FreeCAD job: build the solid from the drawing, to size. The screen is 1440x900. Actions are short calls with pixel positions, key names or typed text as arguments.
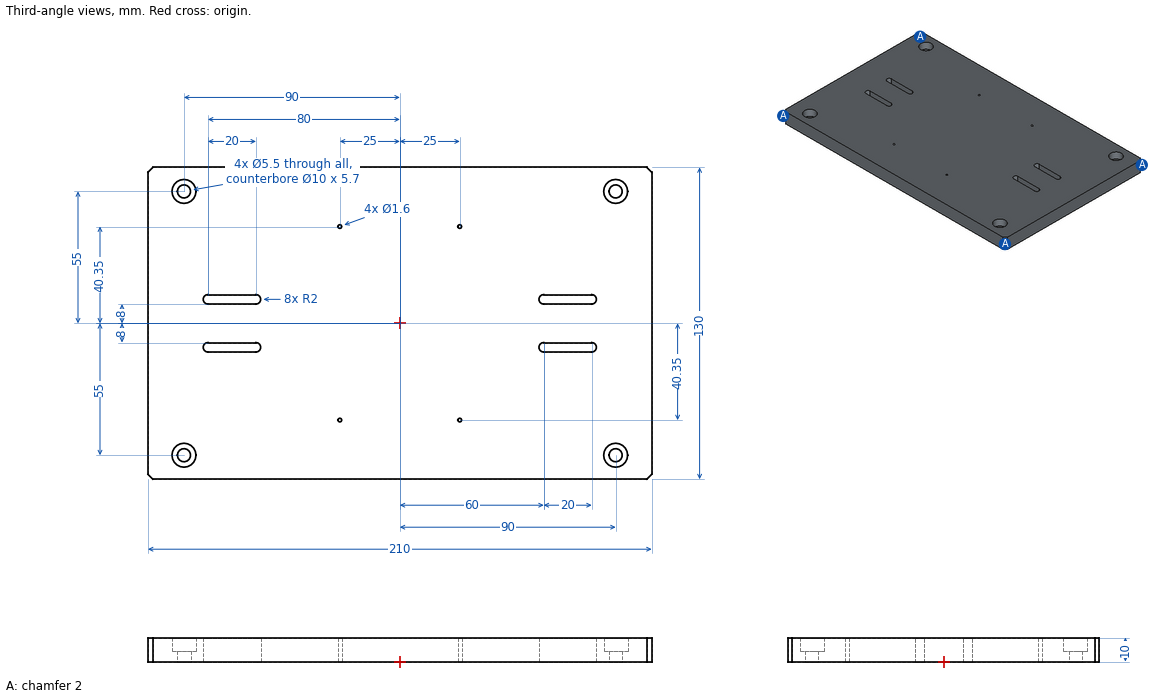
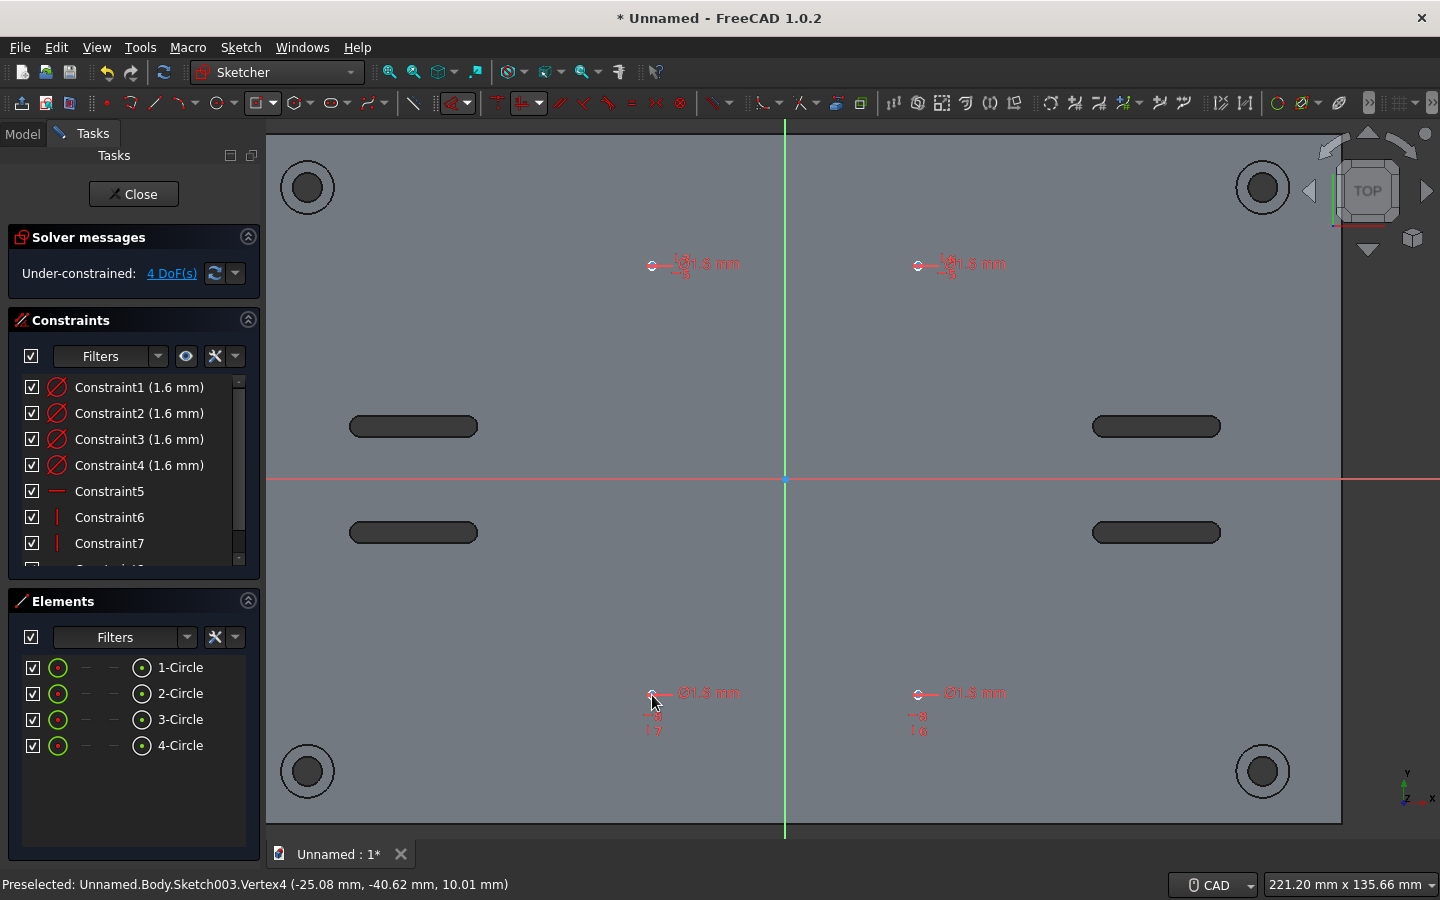
click(652, 266)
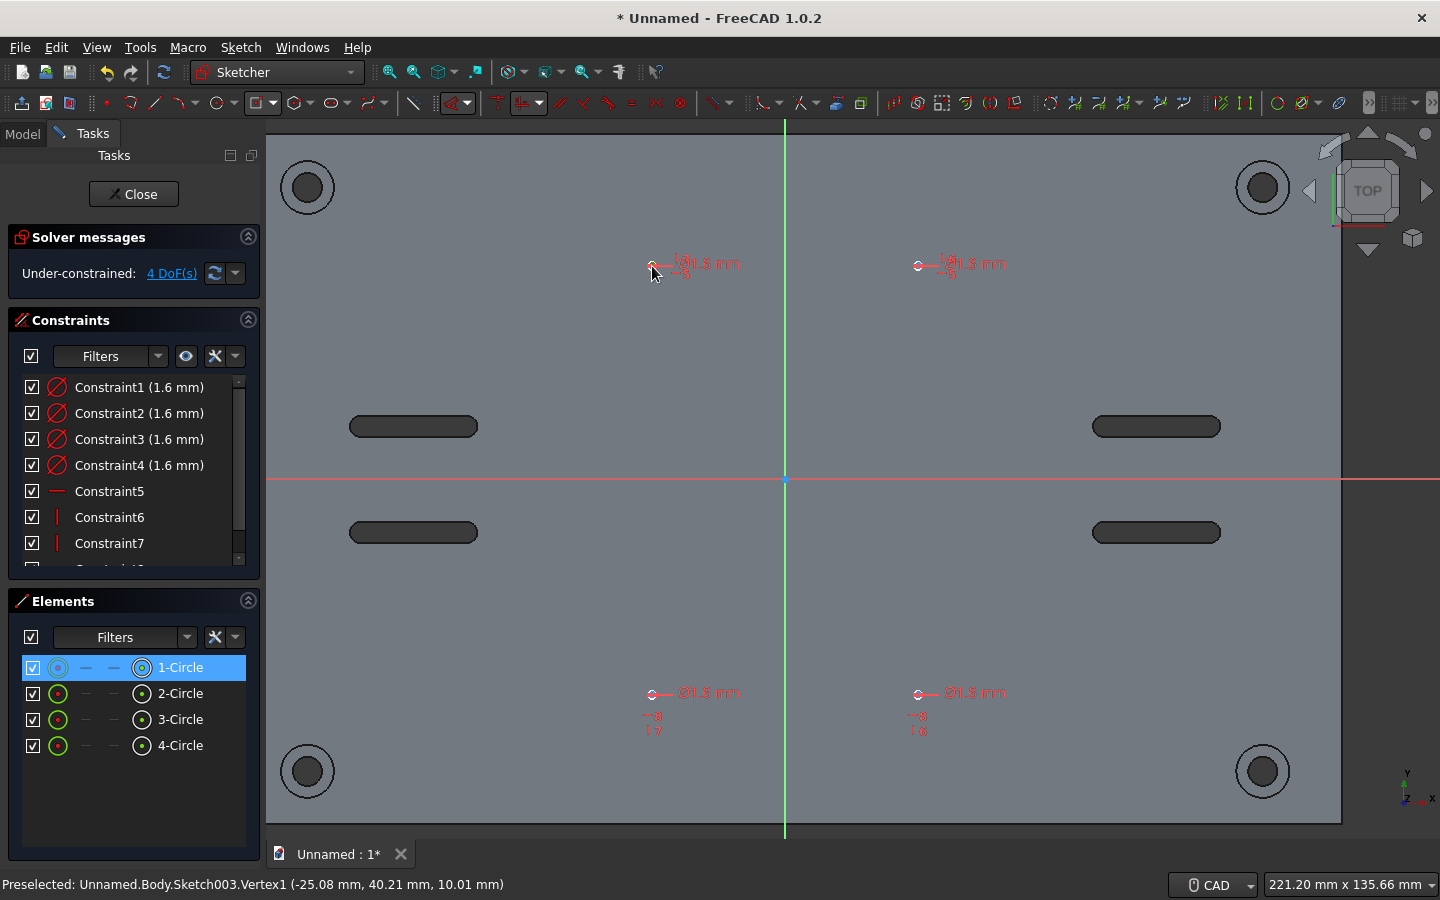
click(470, 104)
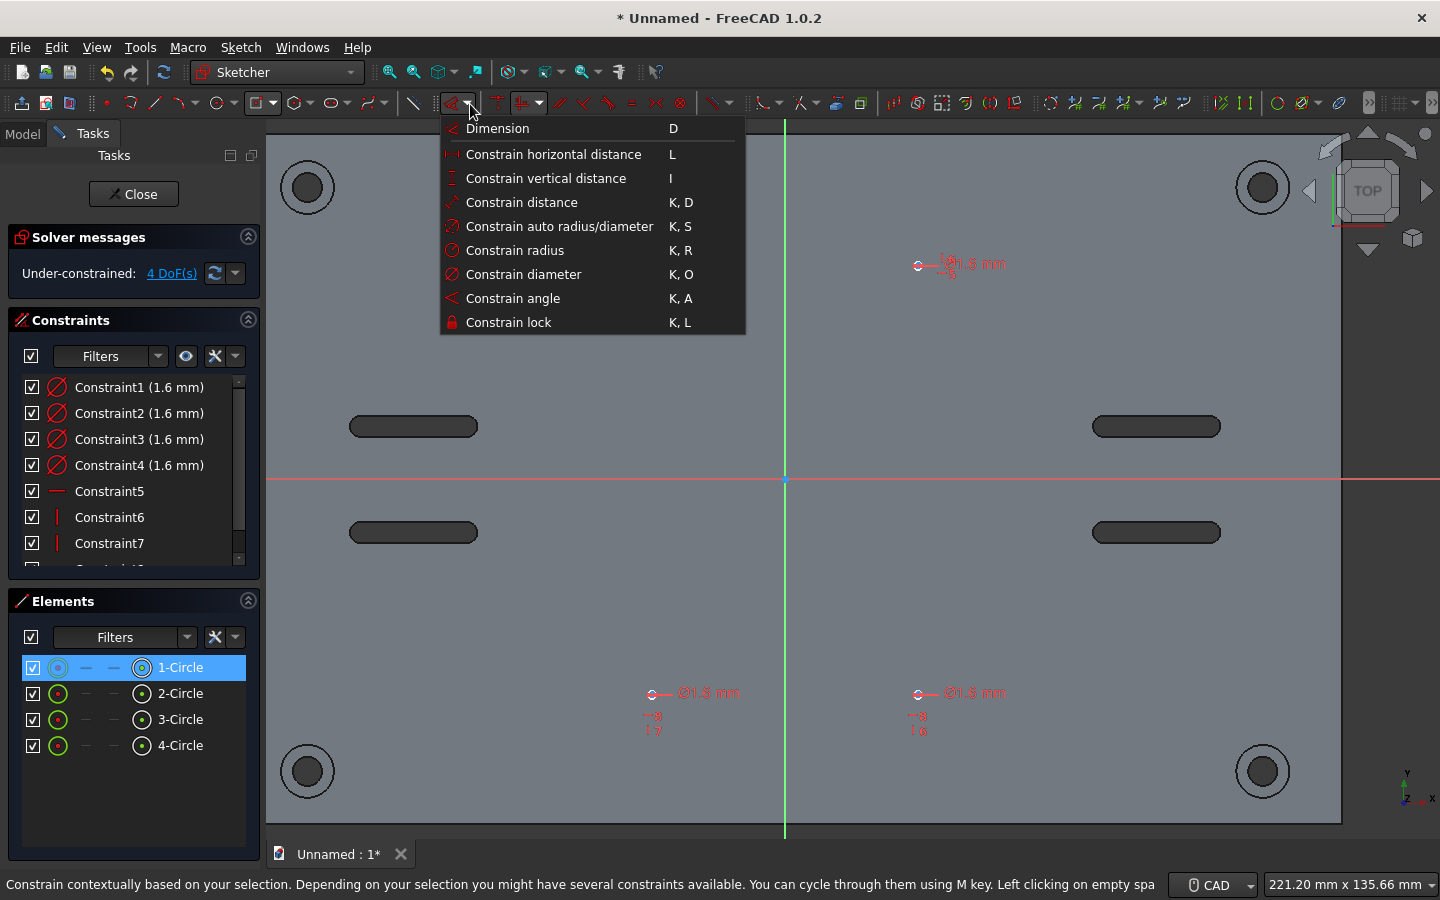
click(593, 154)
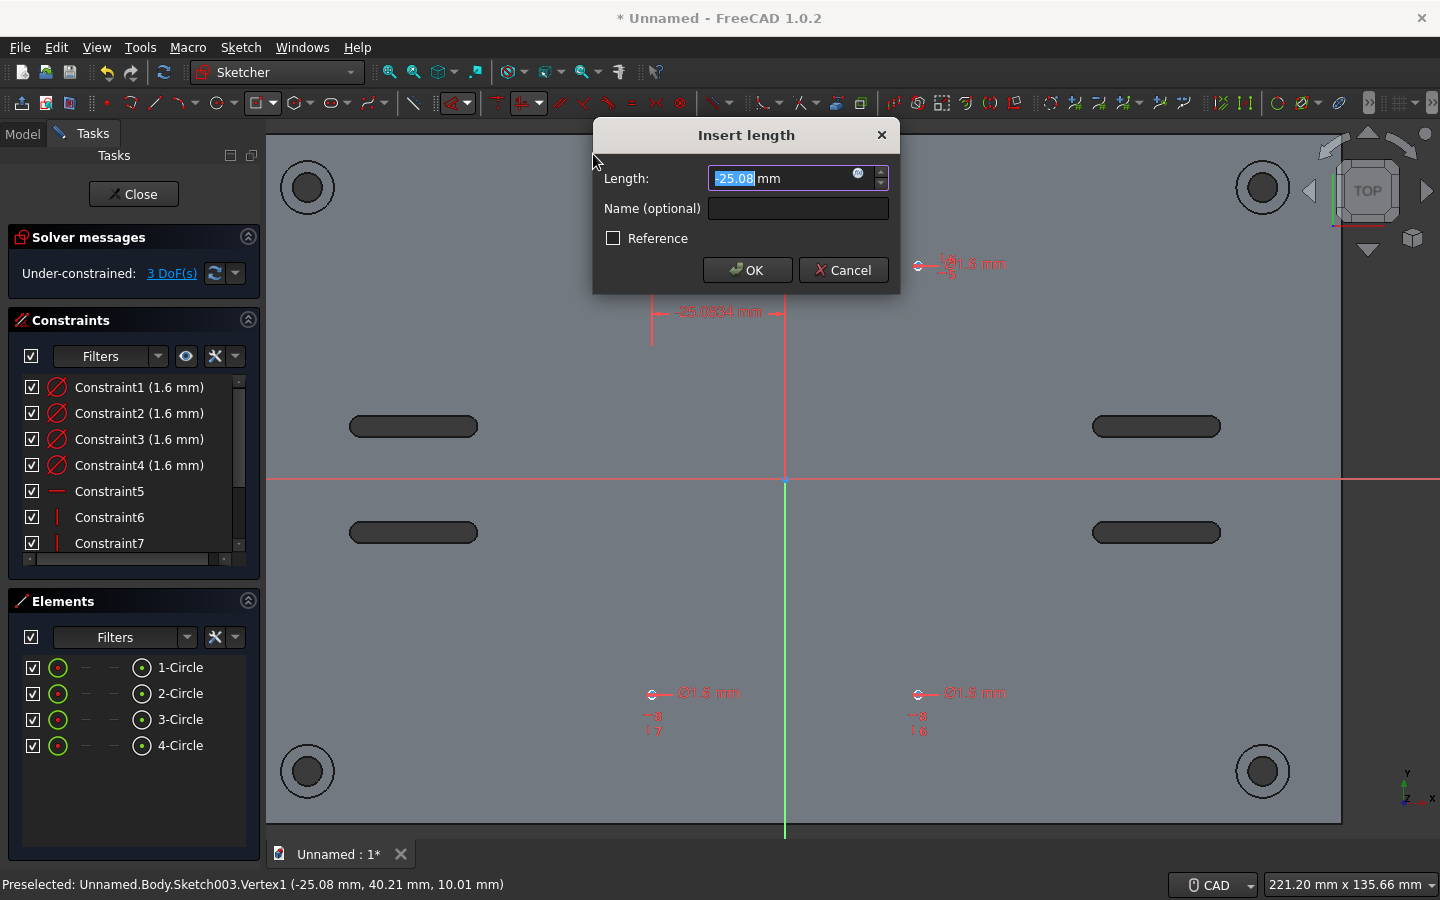
text(-25)
key(Return)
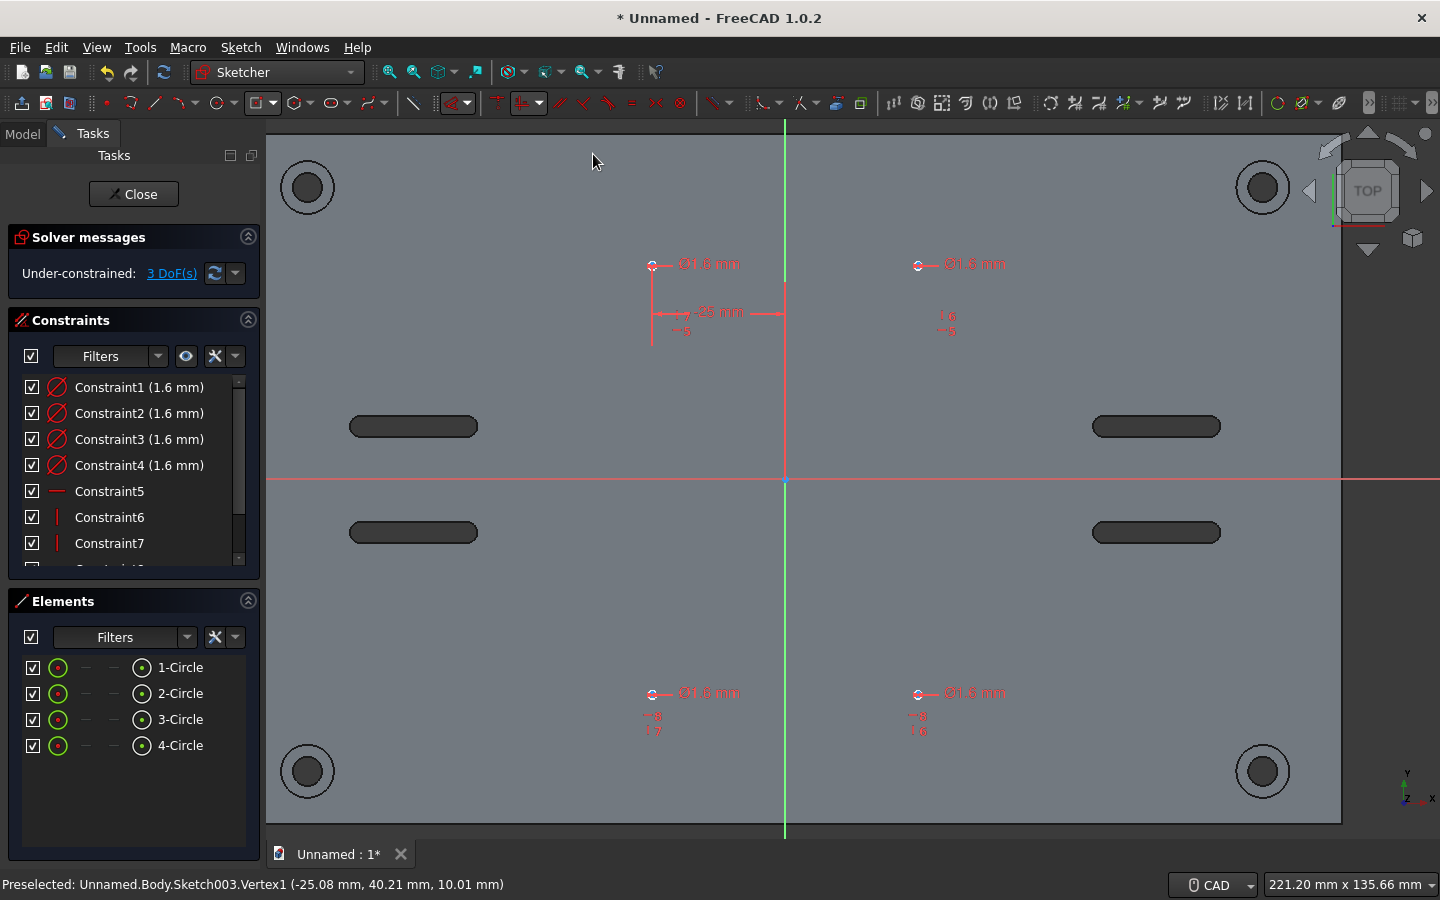
click(918, 266)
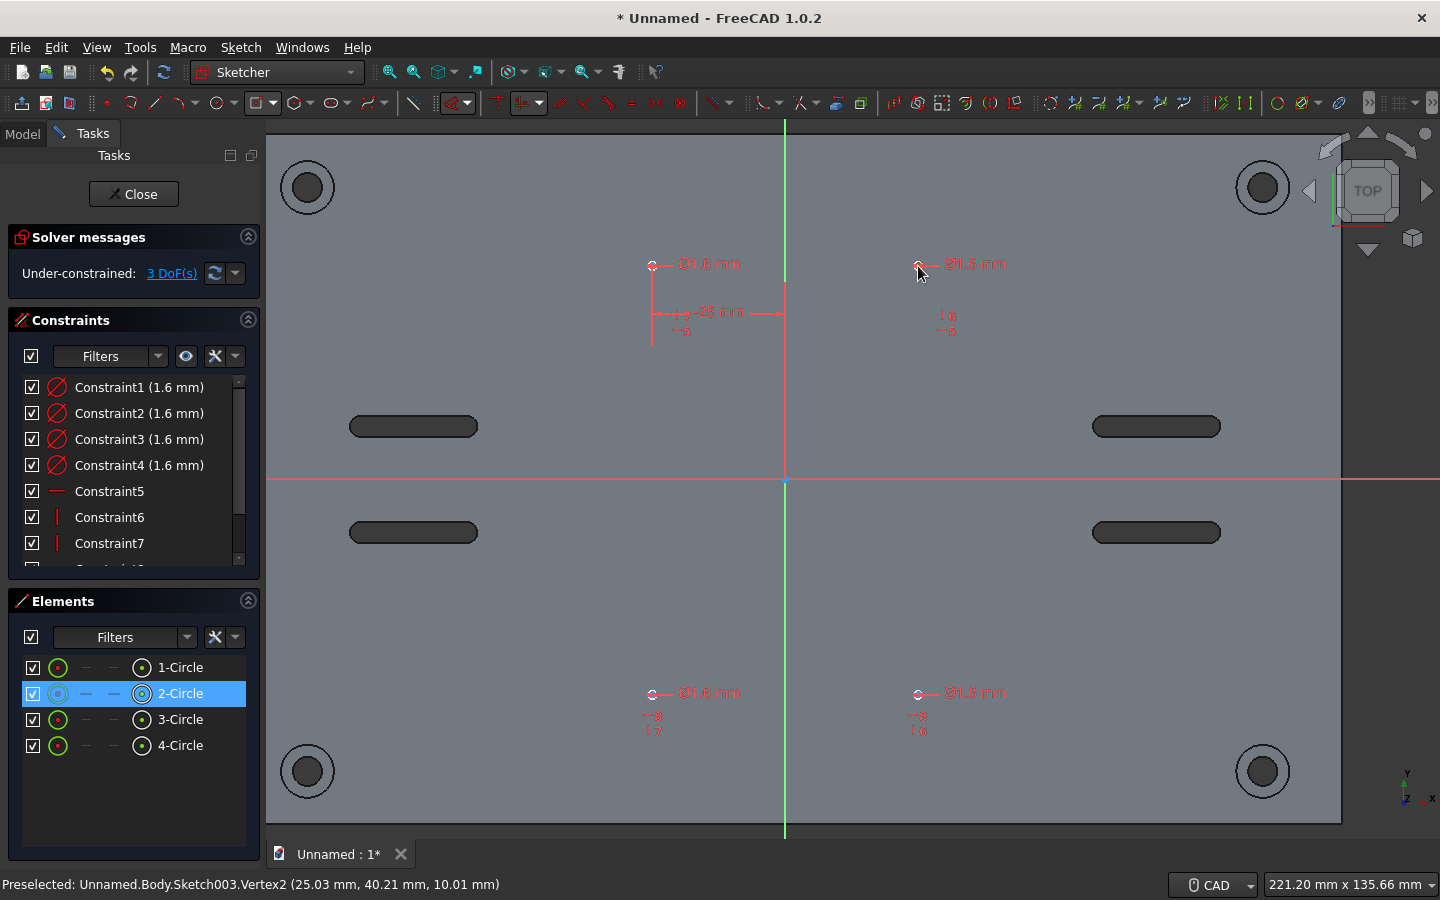
key(l)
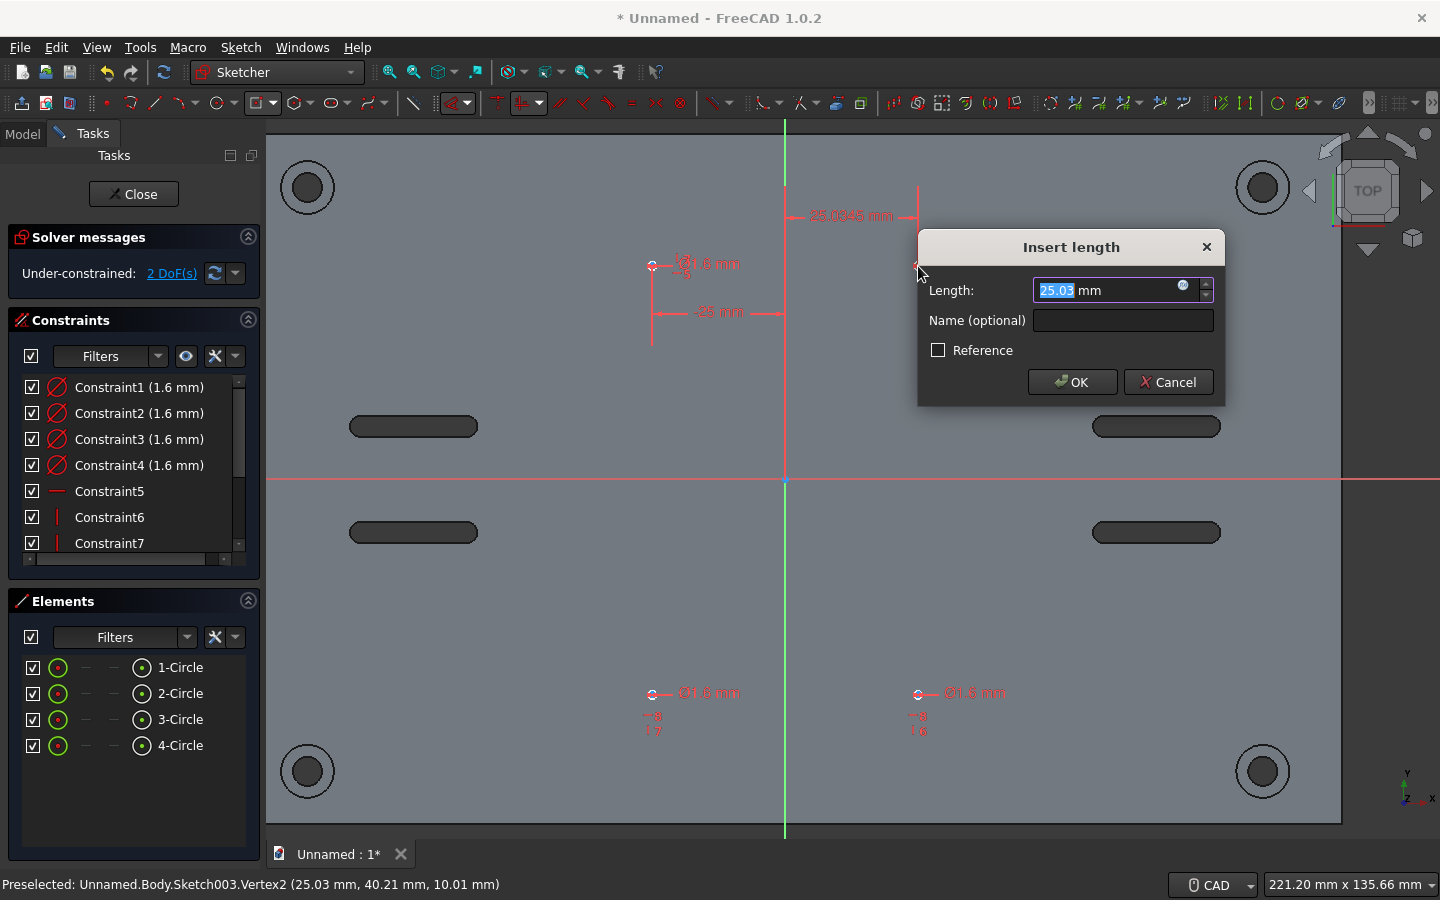
text(25)
key(Return)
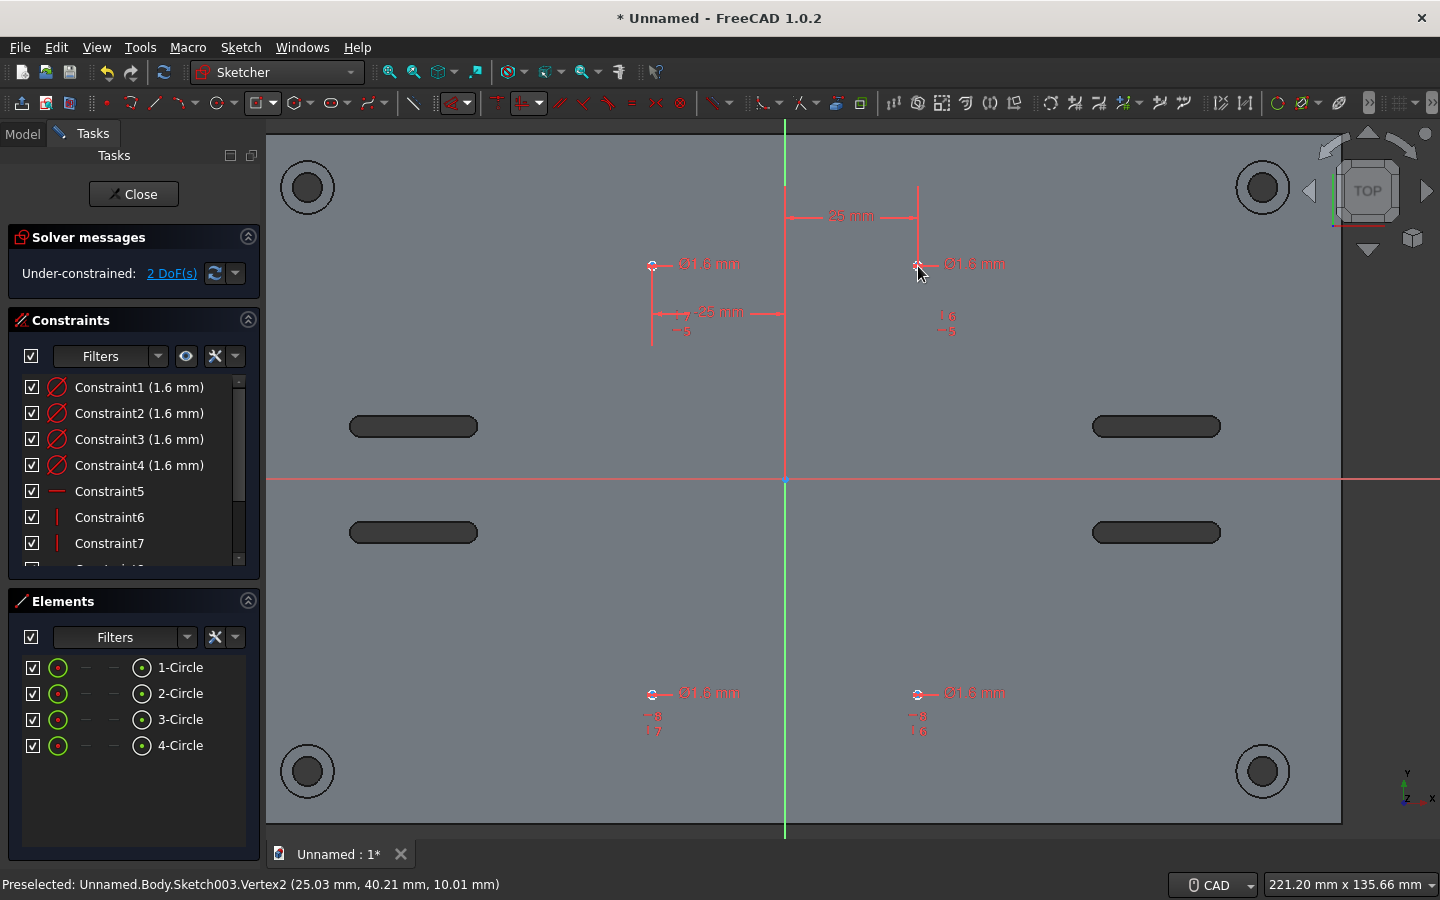
click(652, 266)